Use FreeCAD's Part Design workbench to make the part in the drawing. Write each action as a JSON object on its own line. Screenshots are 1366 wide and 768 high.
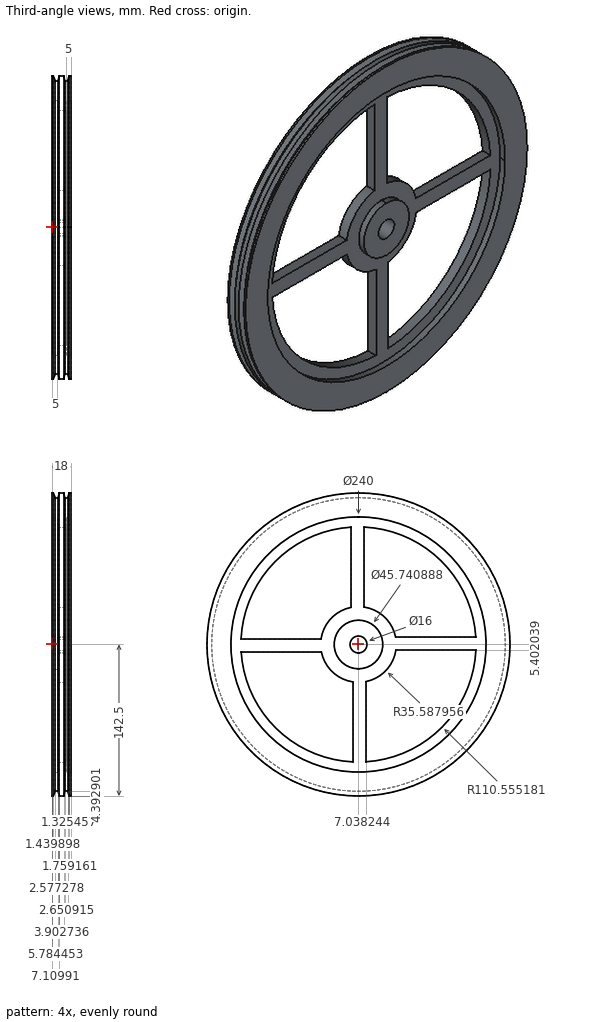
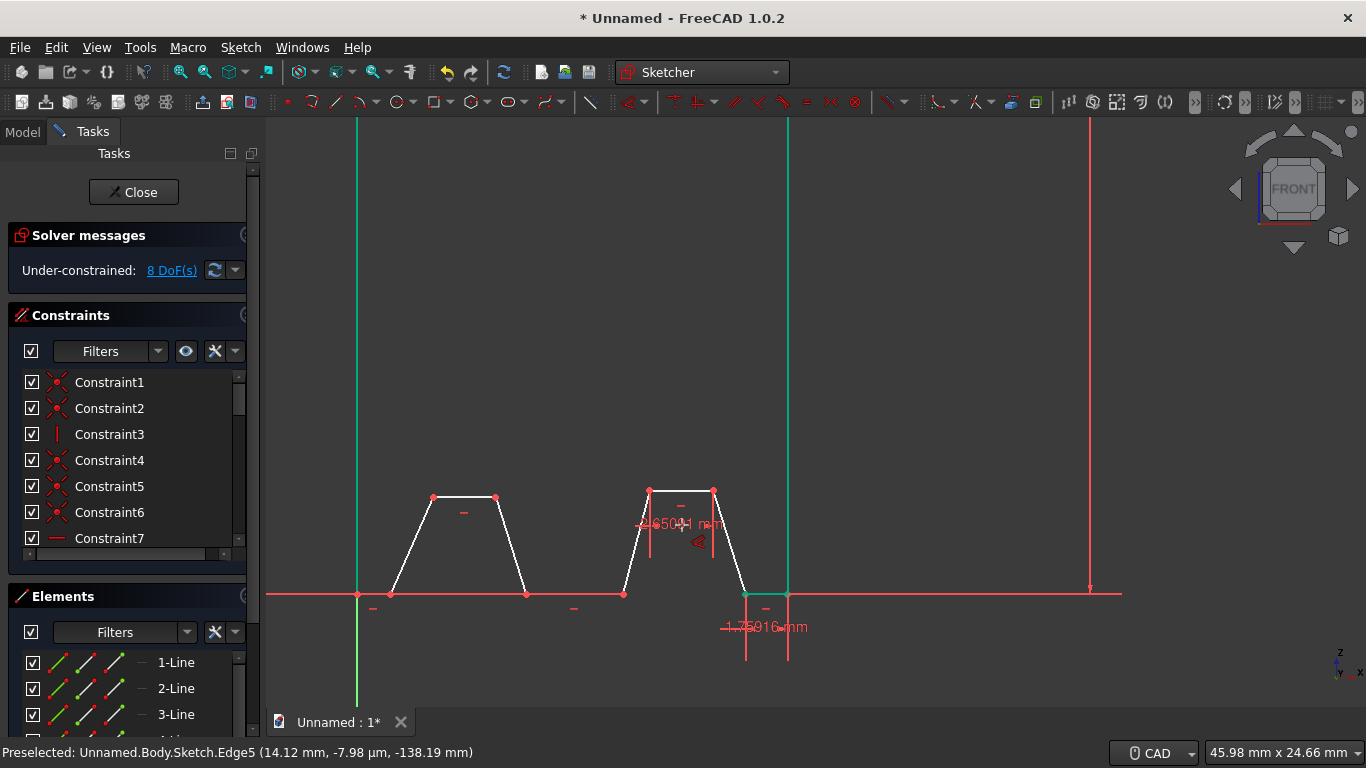
{"action": "left_click", "coordinate": [594, 594]}
{"action": "left_click", "coordinate": [575, 628]}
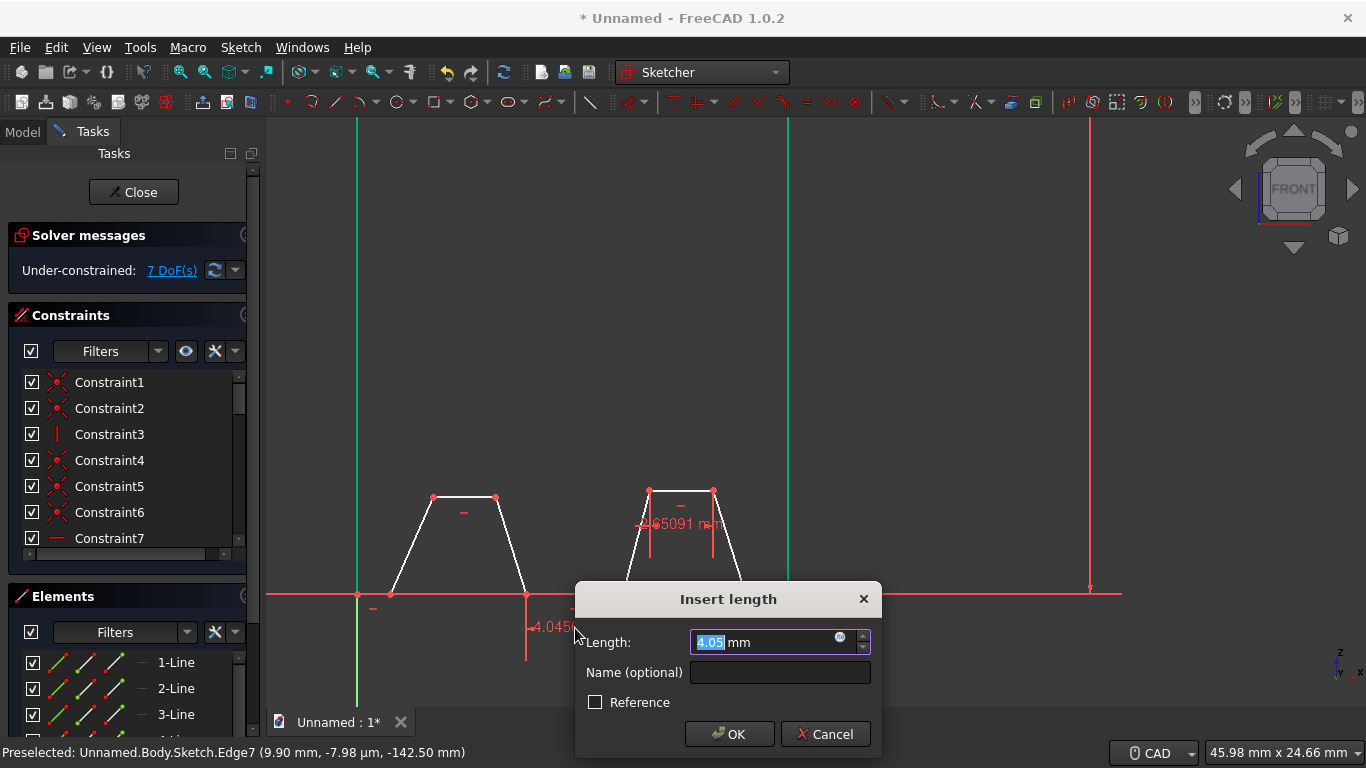
{"action": "type", "text": "3.902736"}
{"action": "key", "text": "Return"}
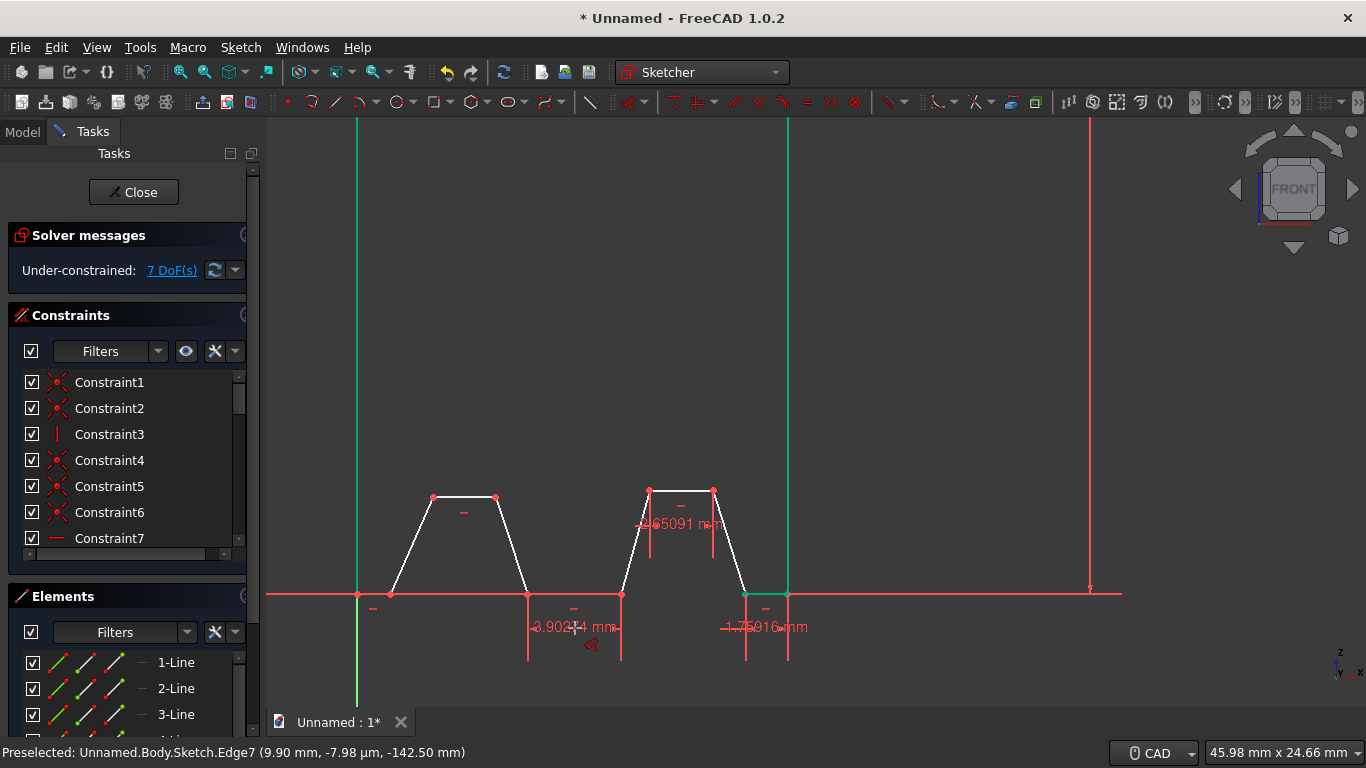
{"action": "left_click", "coordinate": [477, 497]}
{"action": "left_click", "coordinate": [465, 531]}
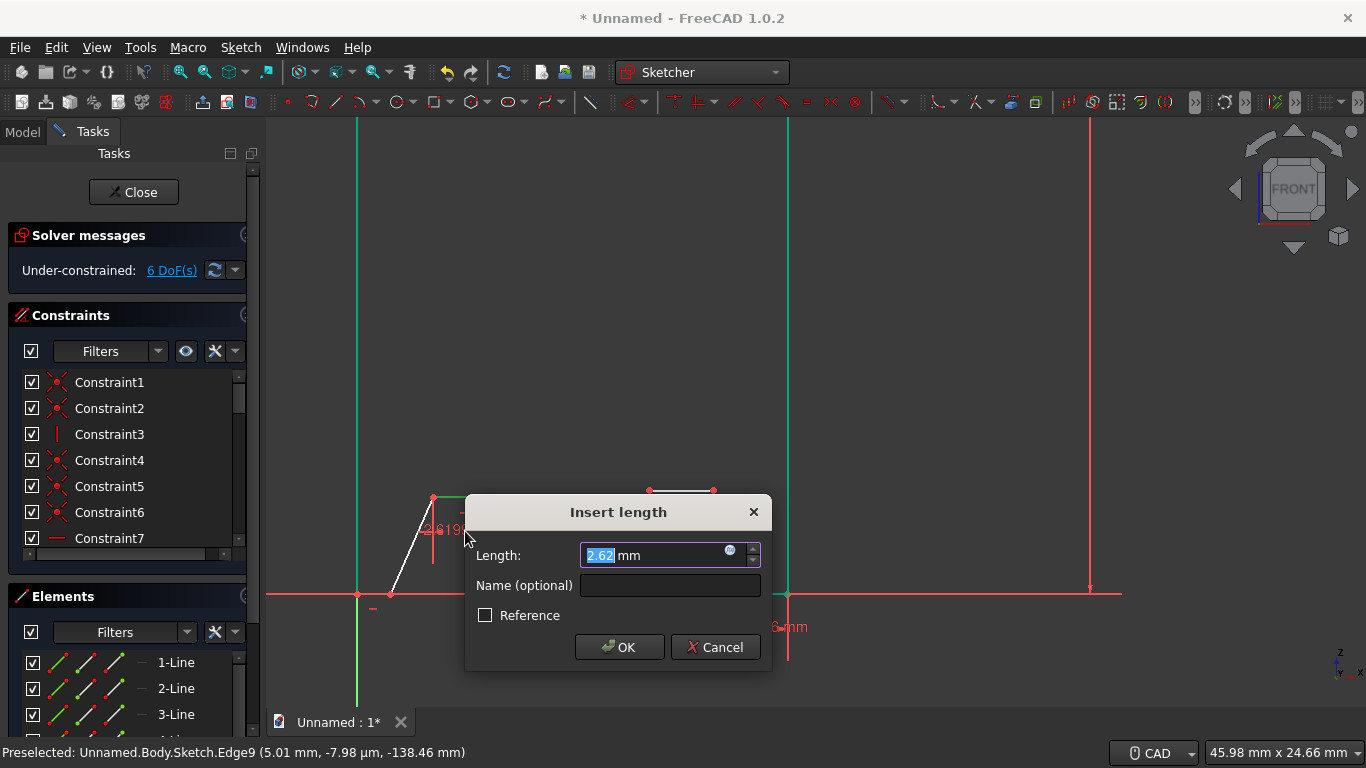
{"action": "type", "text": "2.577278"}
{"action": "key", "text": "Return"}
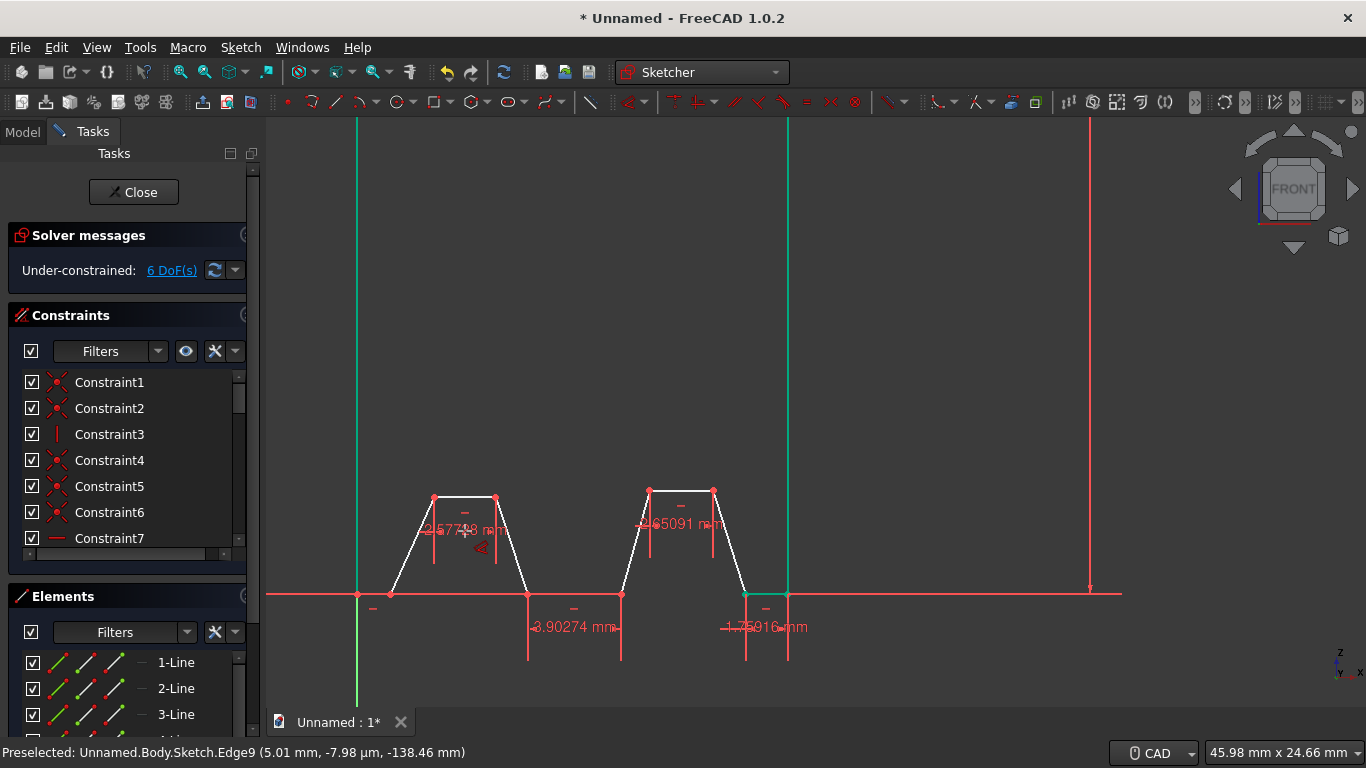
{"action": "scroll", "coordinate": [381, 594], "scroll_direction": "up", "scroll_amount": 2}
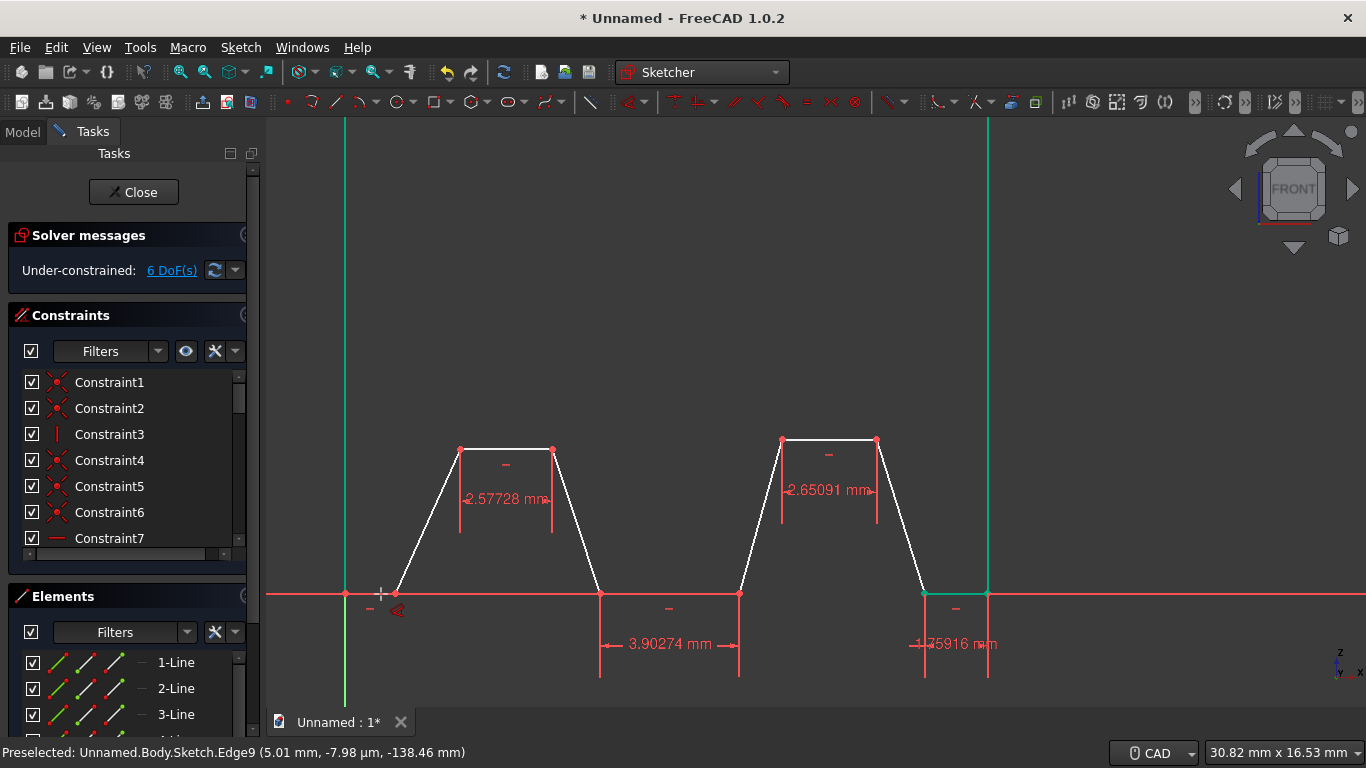
{"action": "left_click", "coordinate": [380, 594]}
{"action": "left_click", "coordinate": [370, 628]}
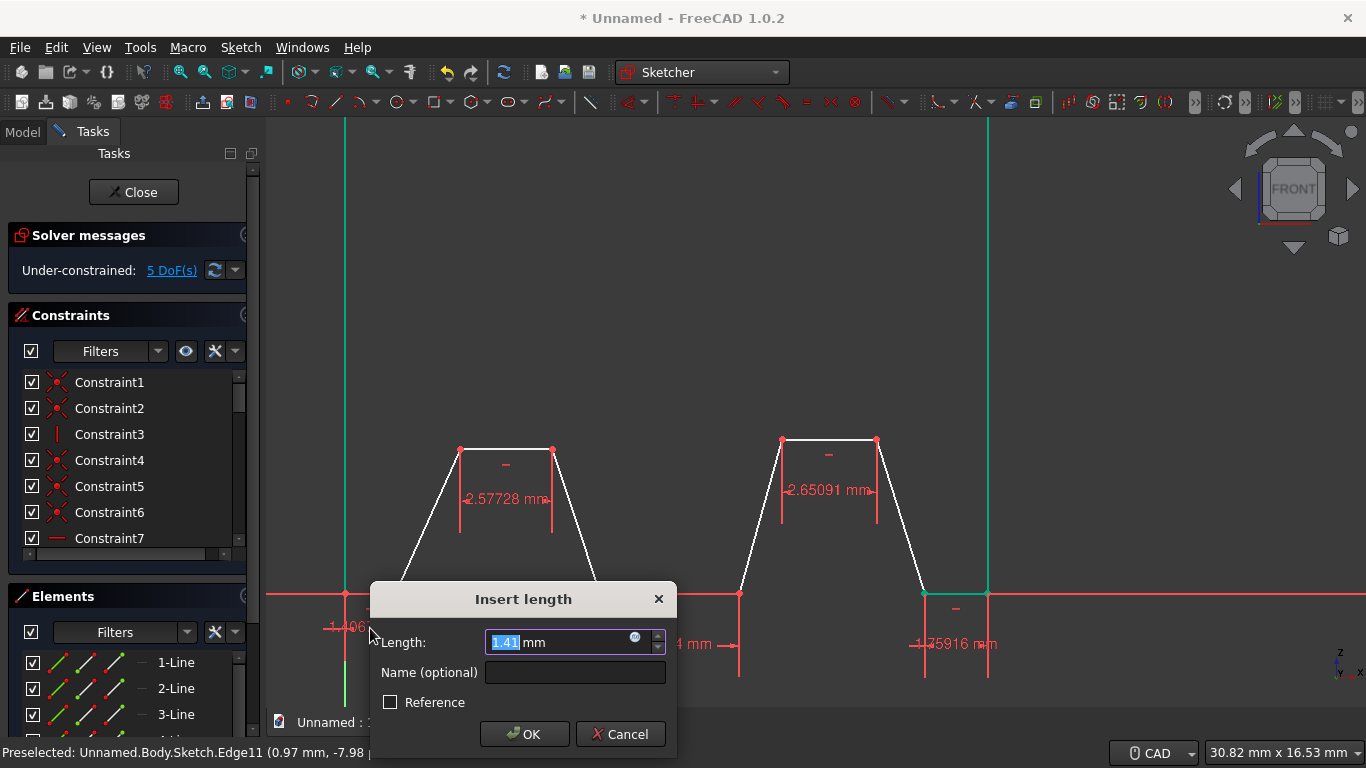
{"action": "type", "text": "1.439898"}
{"action": "key", "text": "Return"}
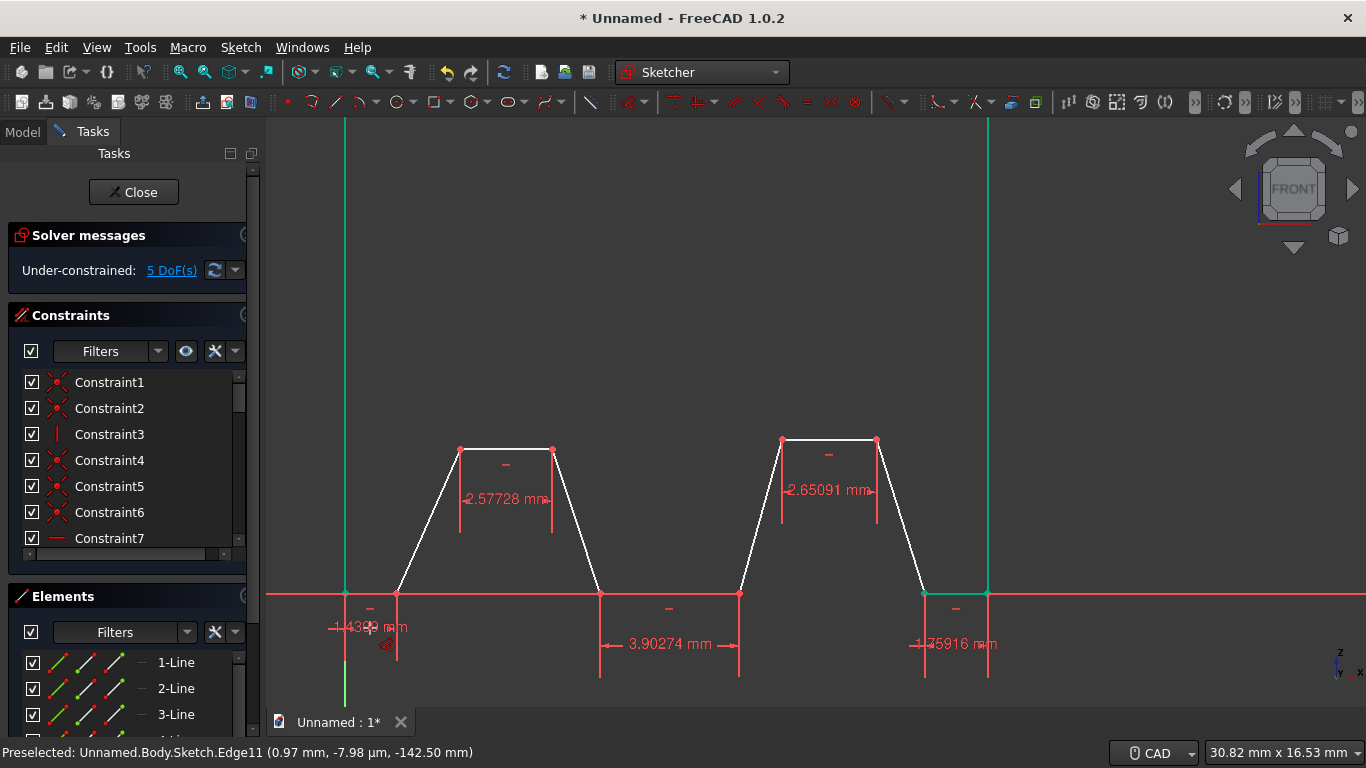
{"action": "scroll", "coordinate": [754, 601], "scroll_direction": "down", "scroll_amount": 13}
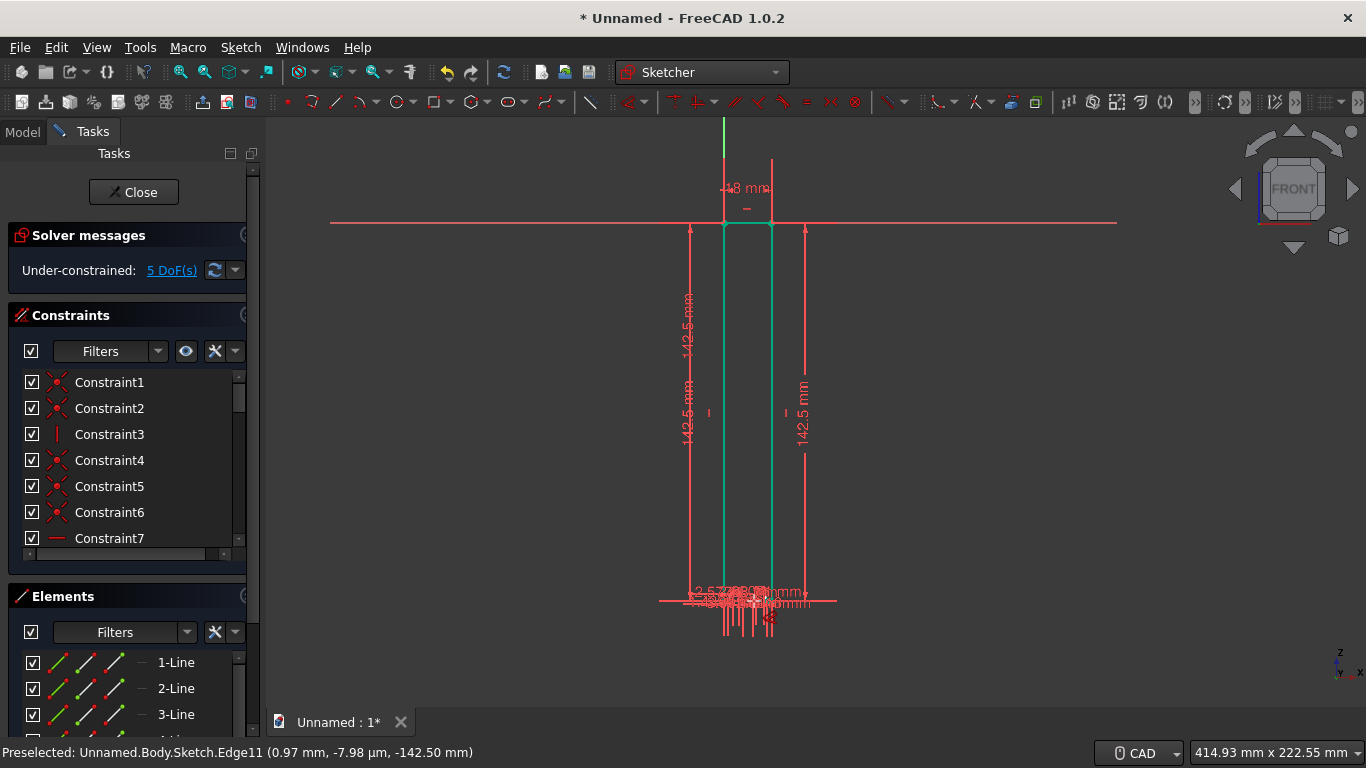
{"action": "scroll", "coordinate": [743, 601], "scroll_direction": "up", "scroll_amount": 4}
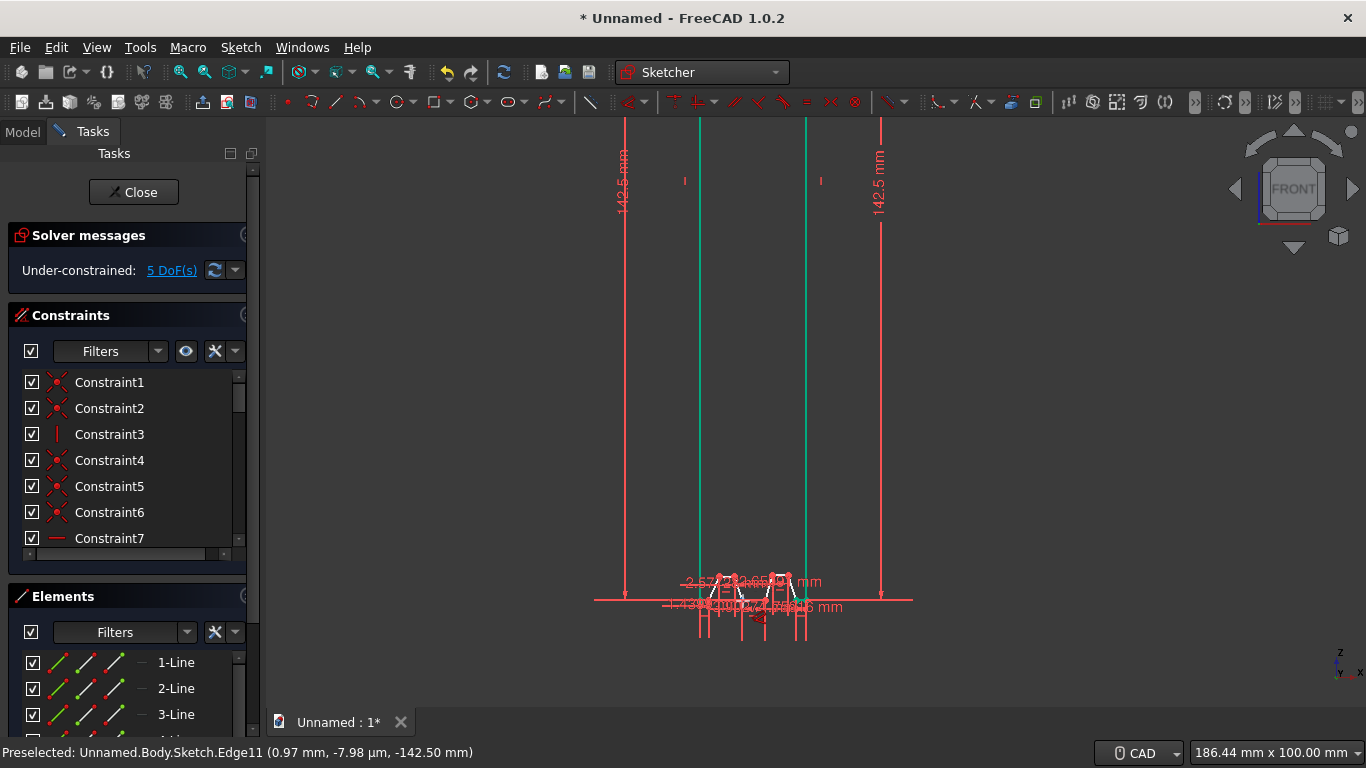
{"action": "left_click", "coordinate": [742, 600]}
{"action": "left_click", "coordinate": [721, 634]}